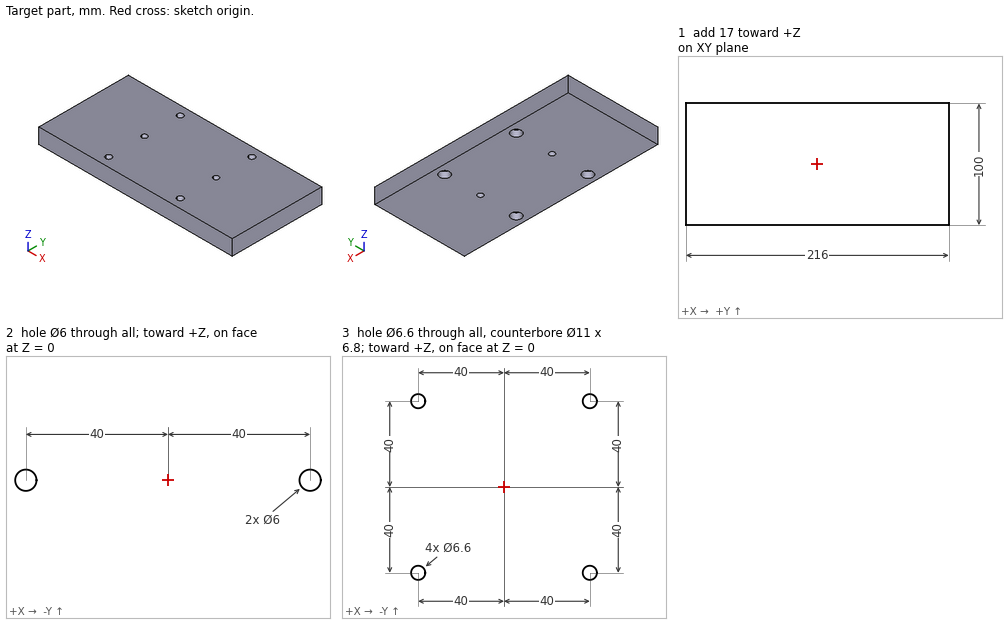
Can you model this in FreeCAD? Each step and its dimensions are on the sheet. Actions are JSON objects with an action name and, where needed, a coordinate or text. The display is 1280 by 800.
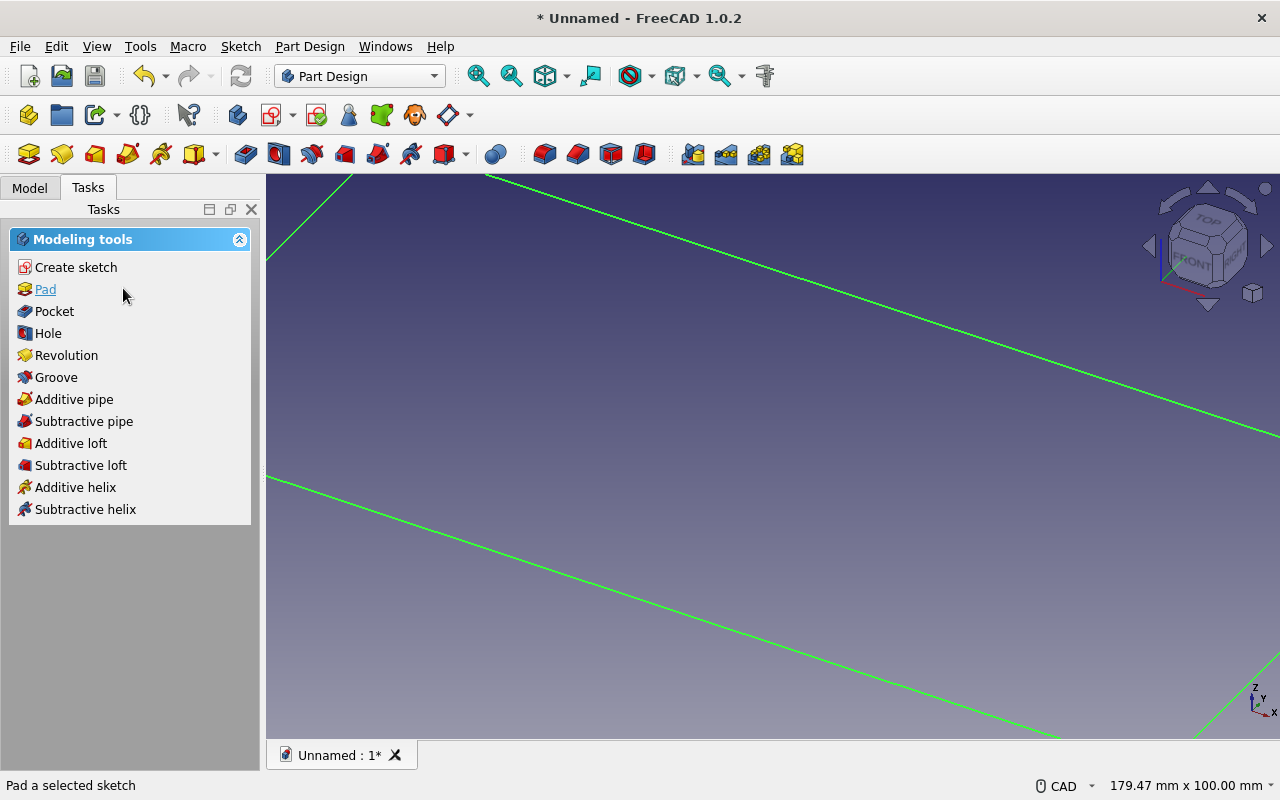
{"action": "left_click", "coordinate": [29, 154]}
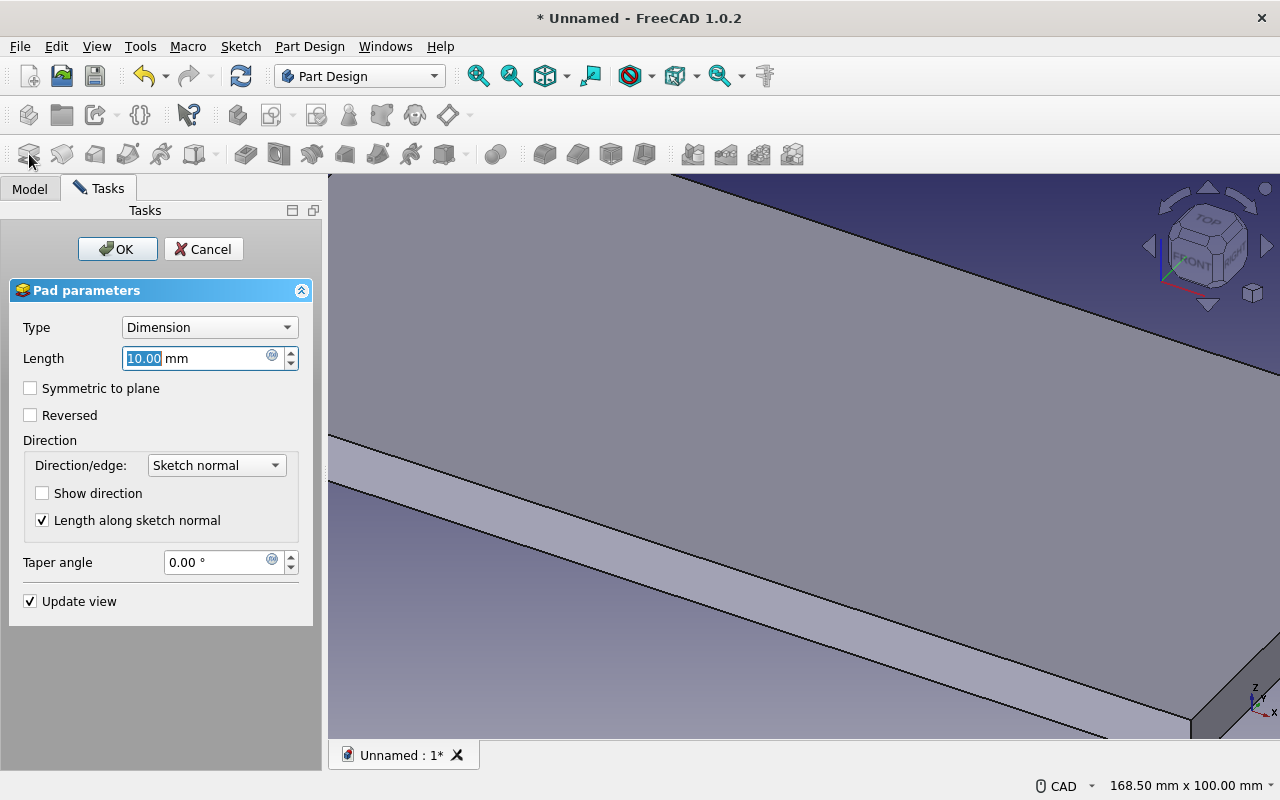
{"action": "type", "text": "17"}
{"action": "key", "text": "Tab"}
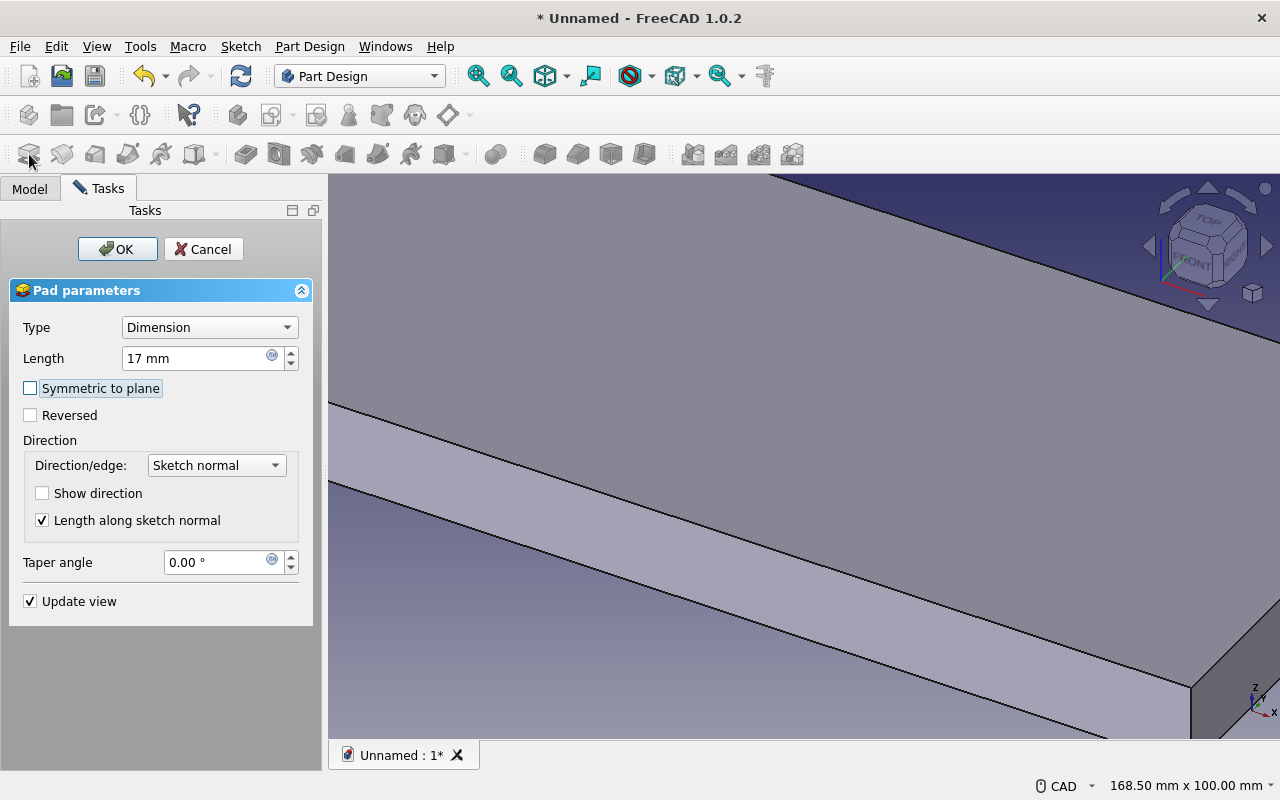
{"action": "left_click", "coordinate": [118, 249]}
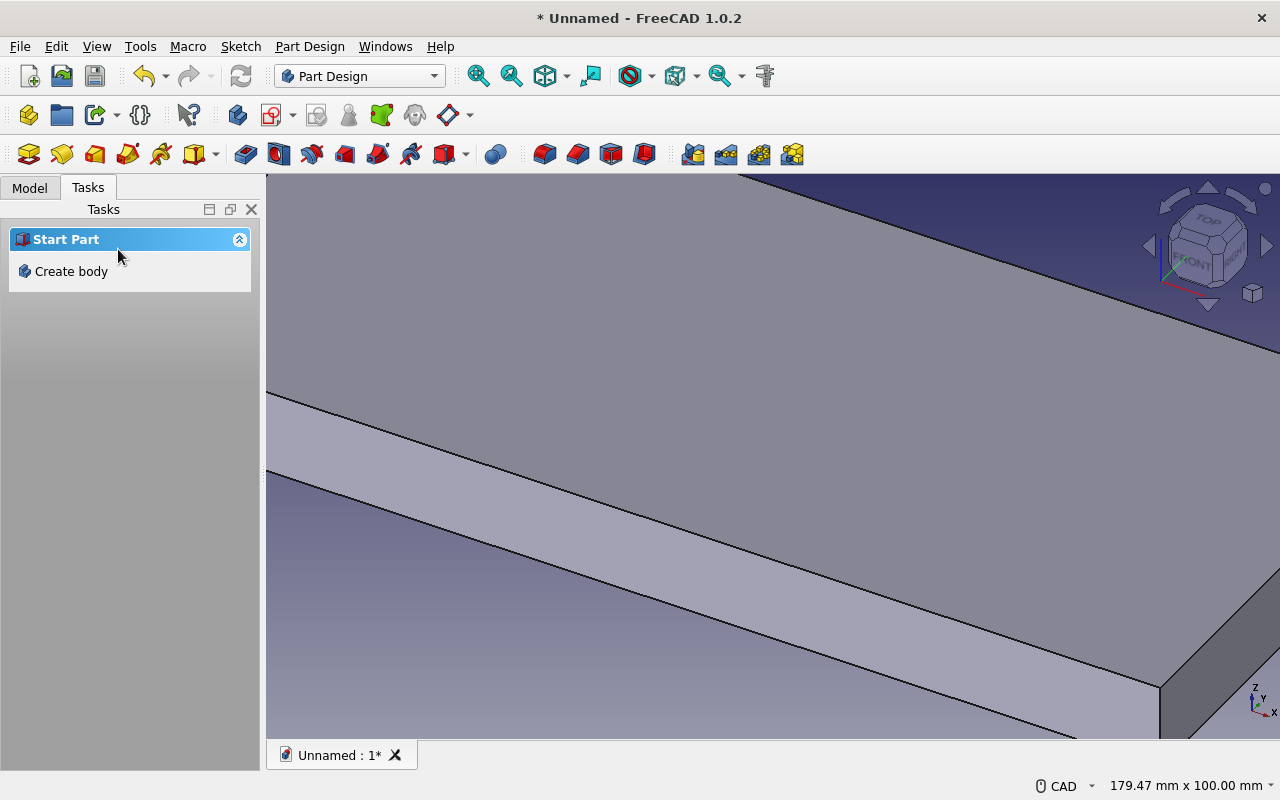
{"action": "left_click", "coordinate": [479, 76]}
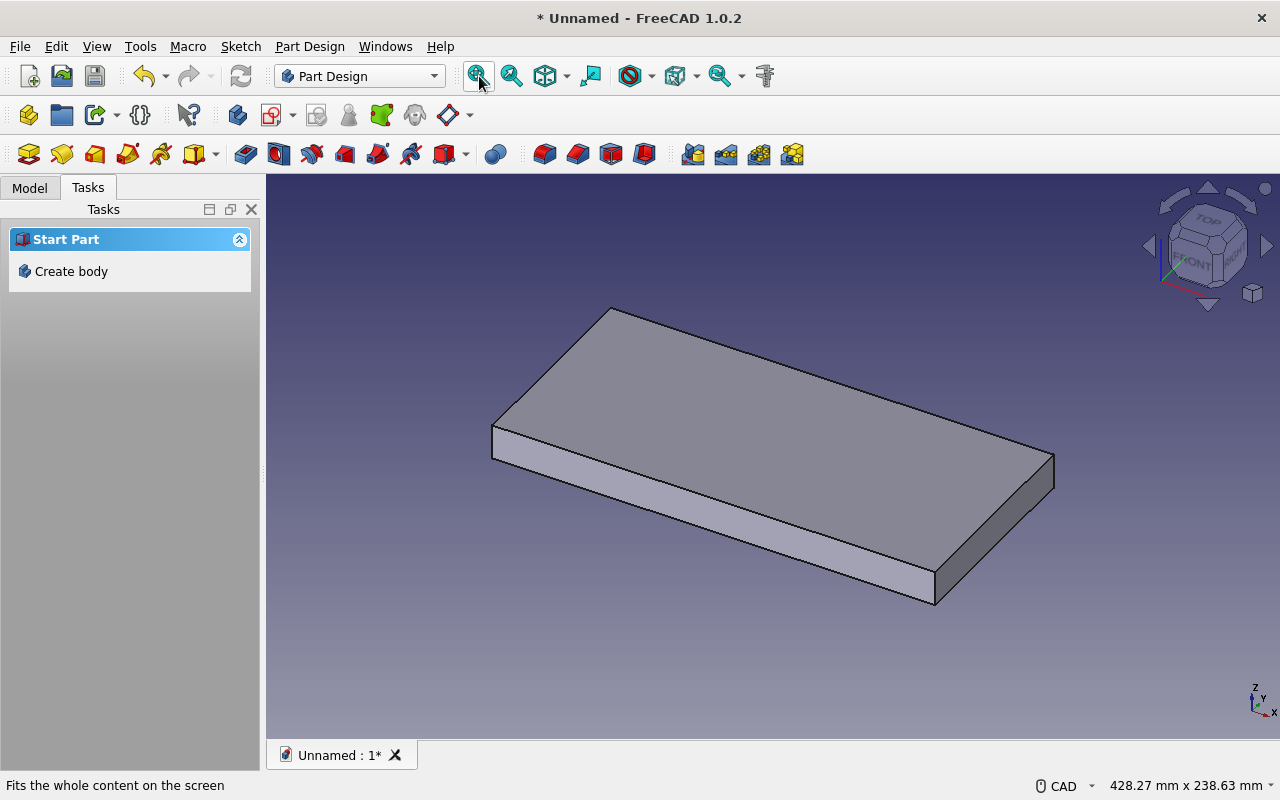
{"action": "key", "text": "5"}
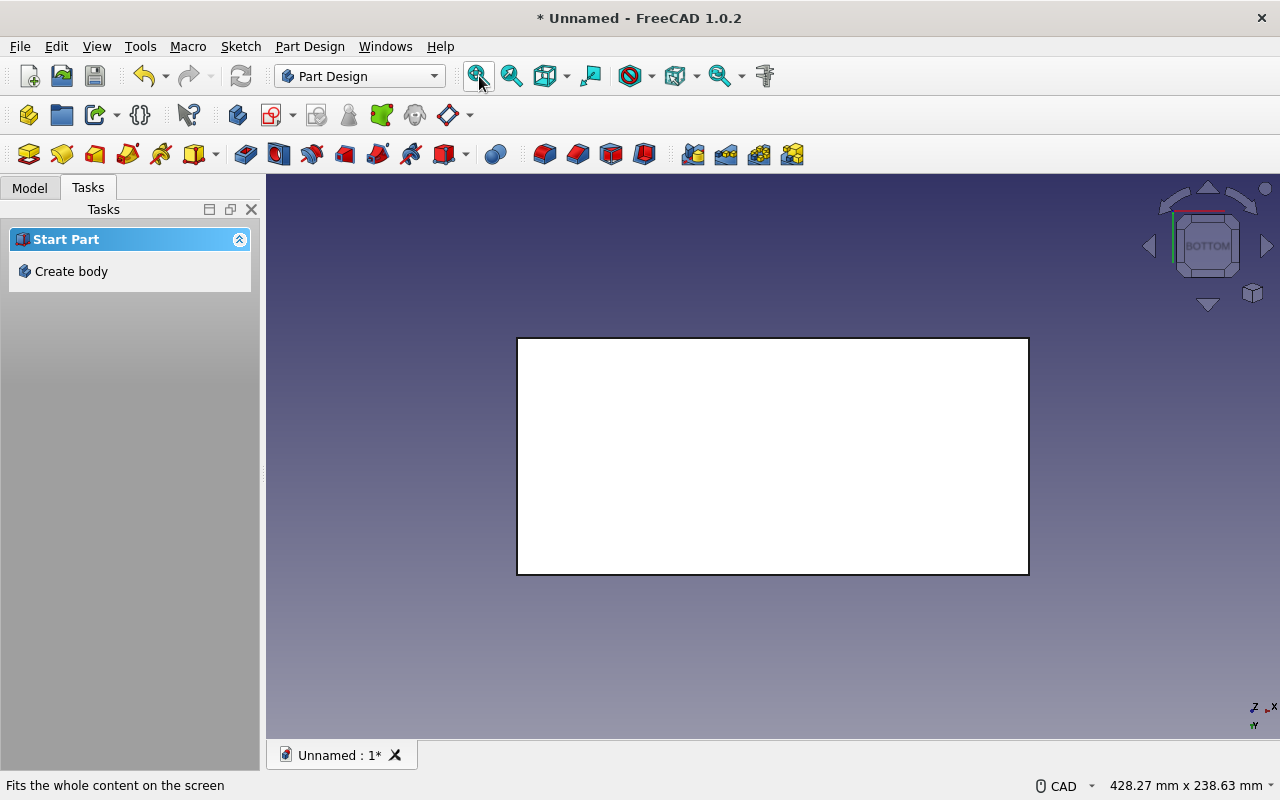
{"action": "left_click", "coordinate": [846, 455]}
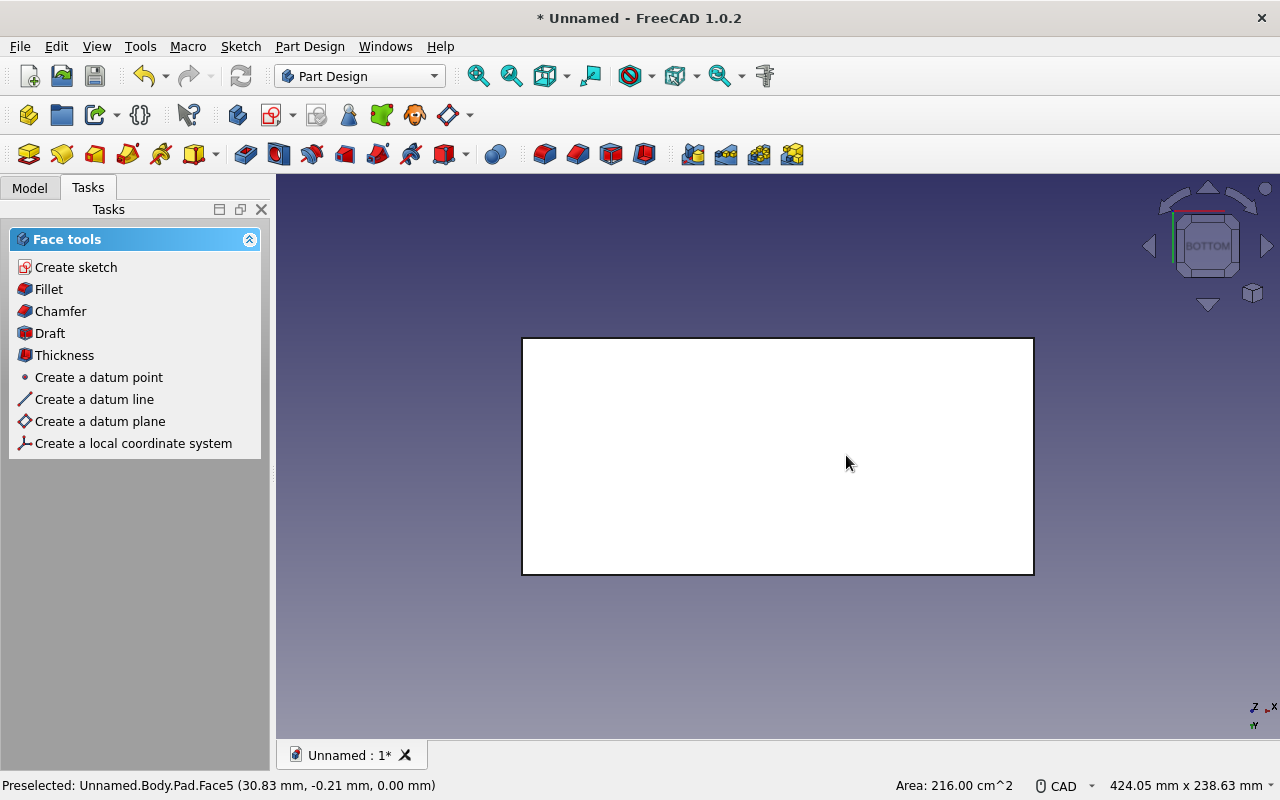
{"action": "left_click", "coordinate": [270, 116]}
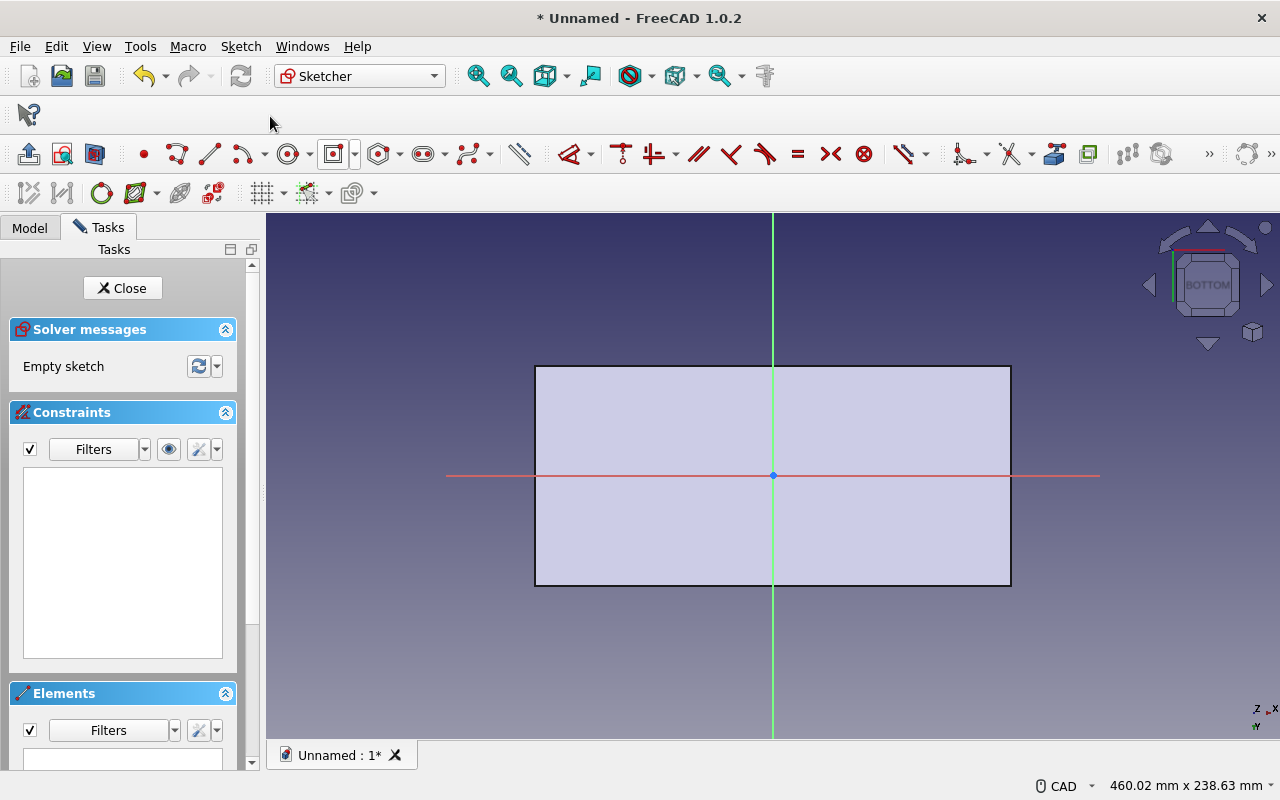
{"action": "scroll", "coordinate": [803, 476], "scroll_direction": "up", "scroll_amount": 6}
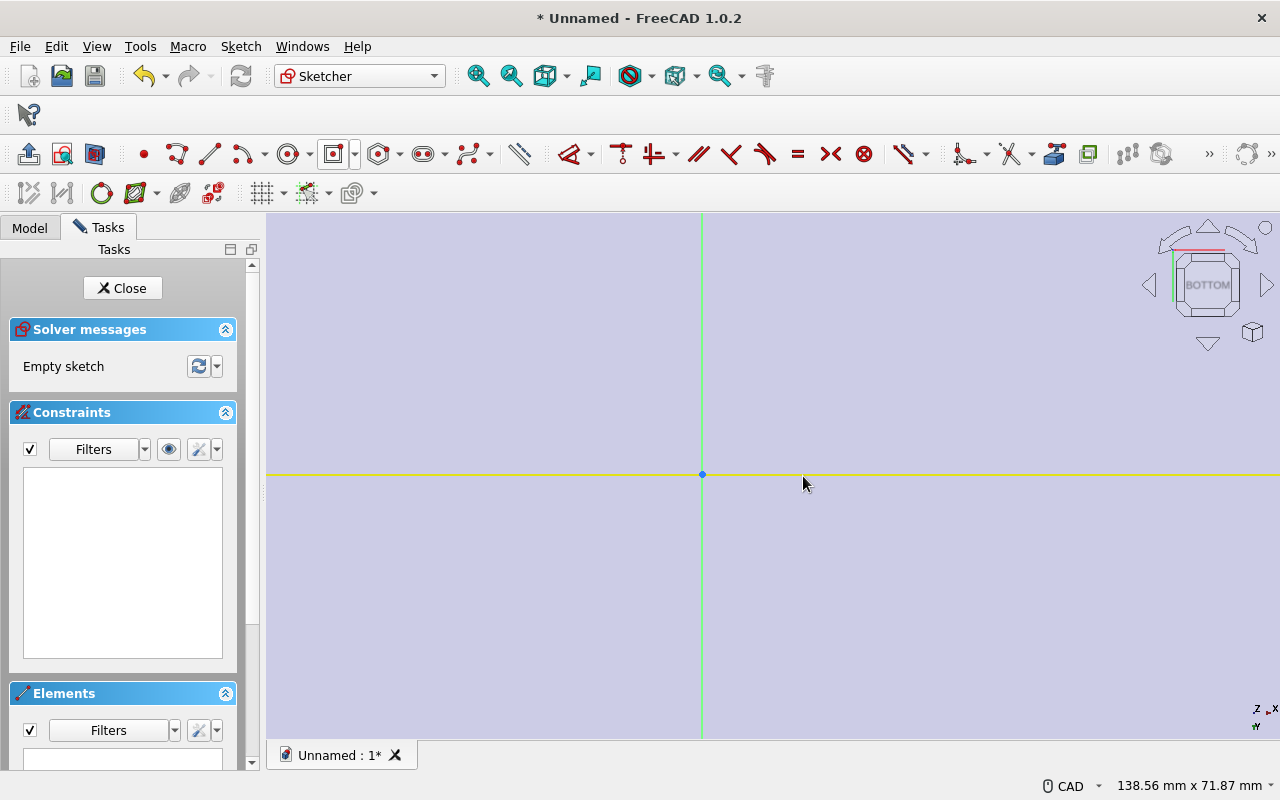
{"action": "left_click", "coordinate": [288, 154]}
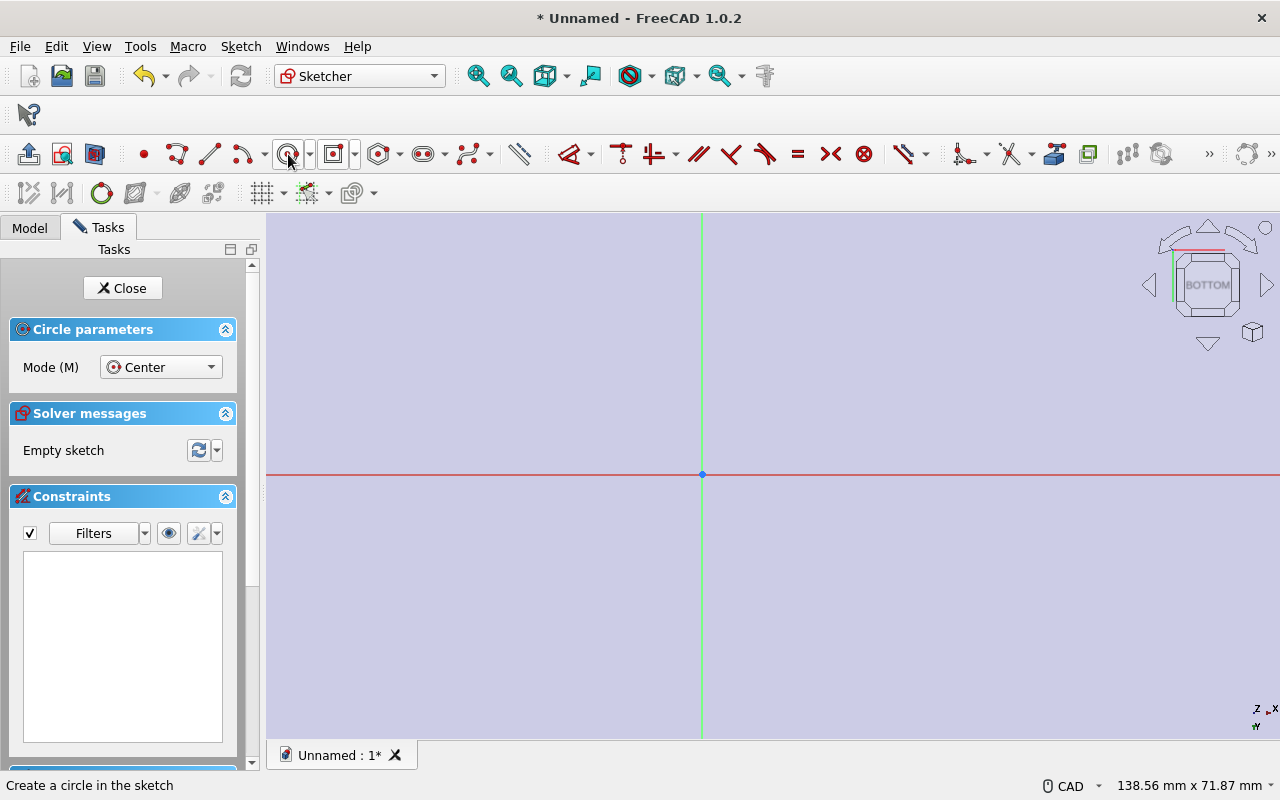
{"action": "left_click", "coordinate": [995, 475]}
{"action": "mouse_move", "coordinate": [1010, 459]}